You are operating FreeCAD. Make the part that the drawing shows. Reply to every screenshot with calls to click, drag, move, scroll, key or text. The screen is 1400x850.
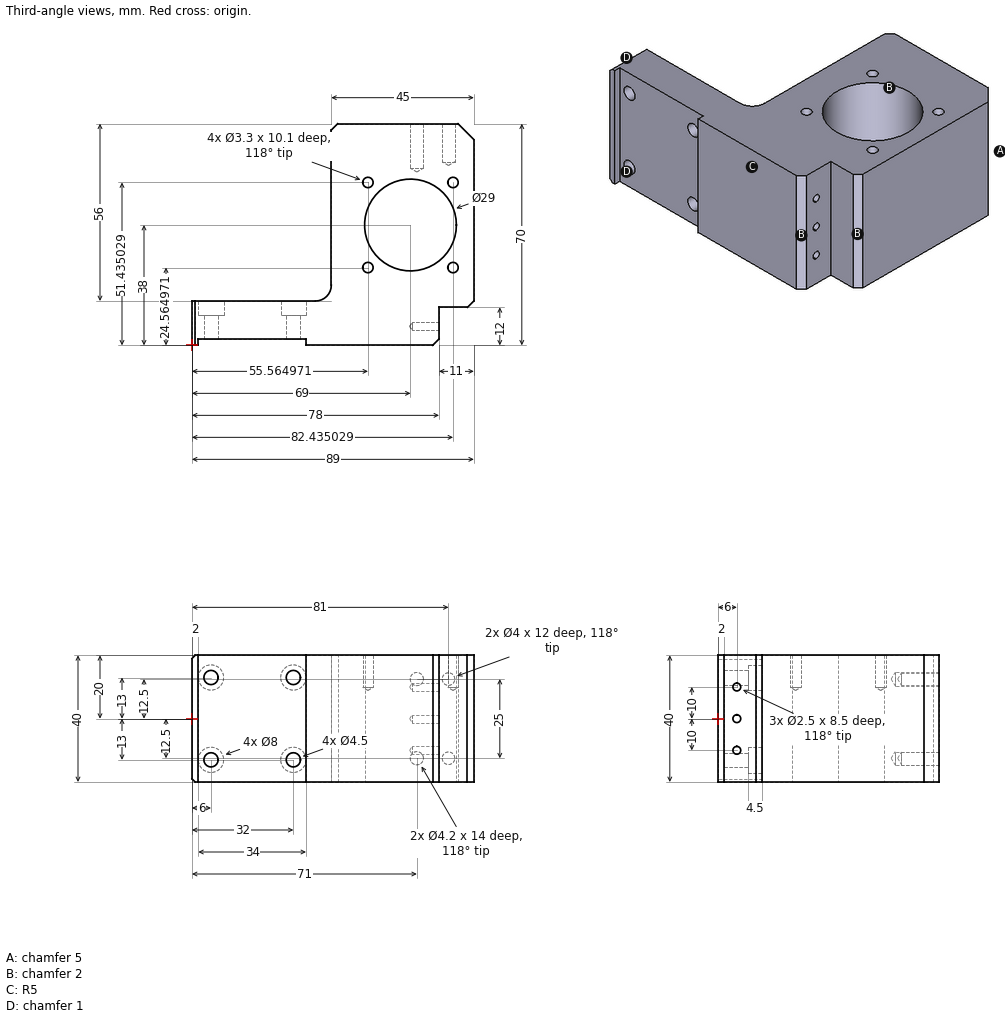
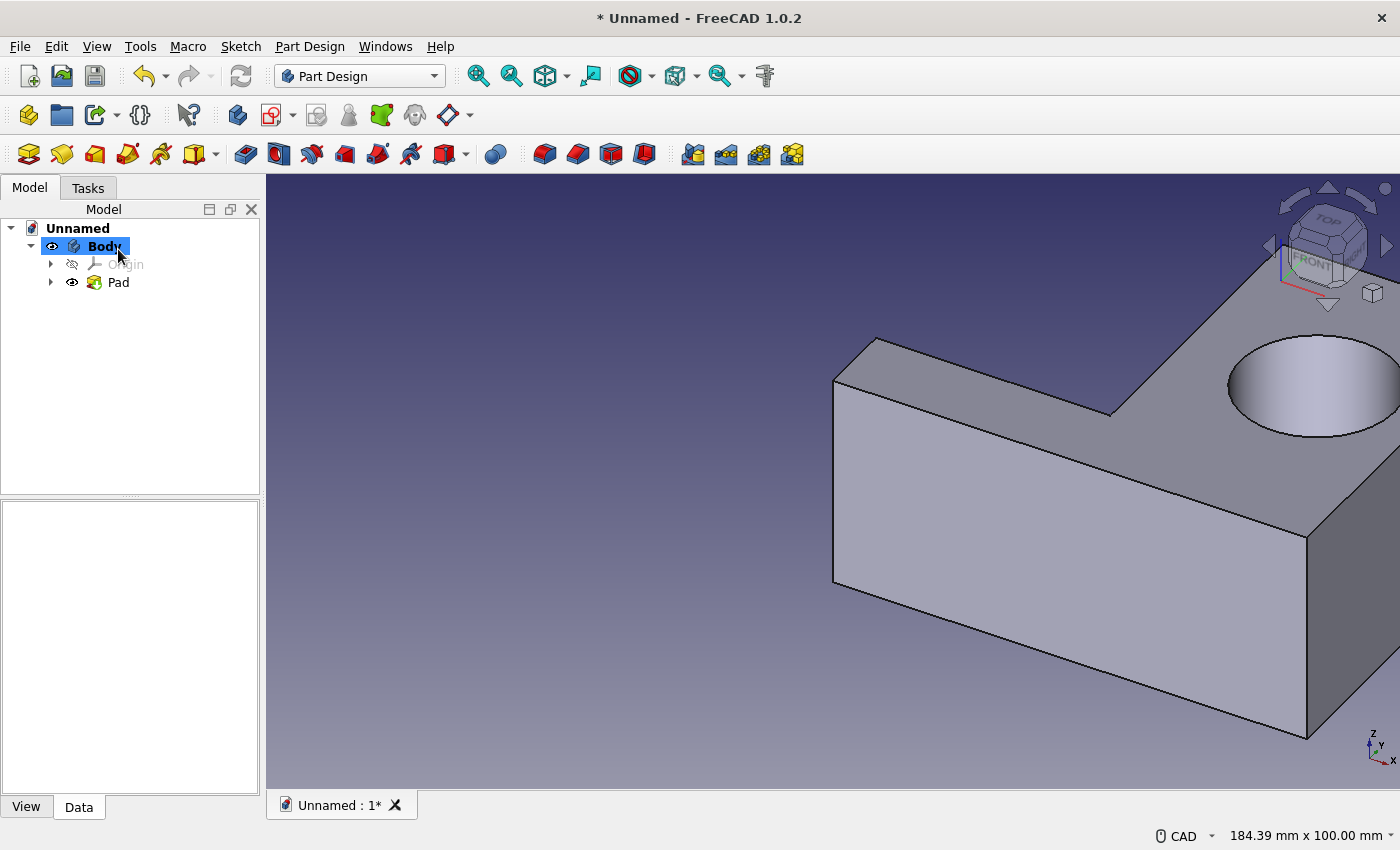
click(479, 76)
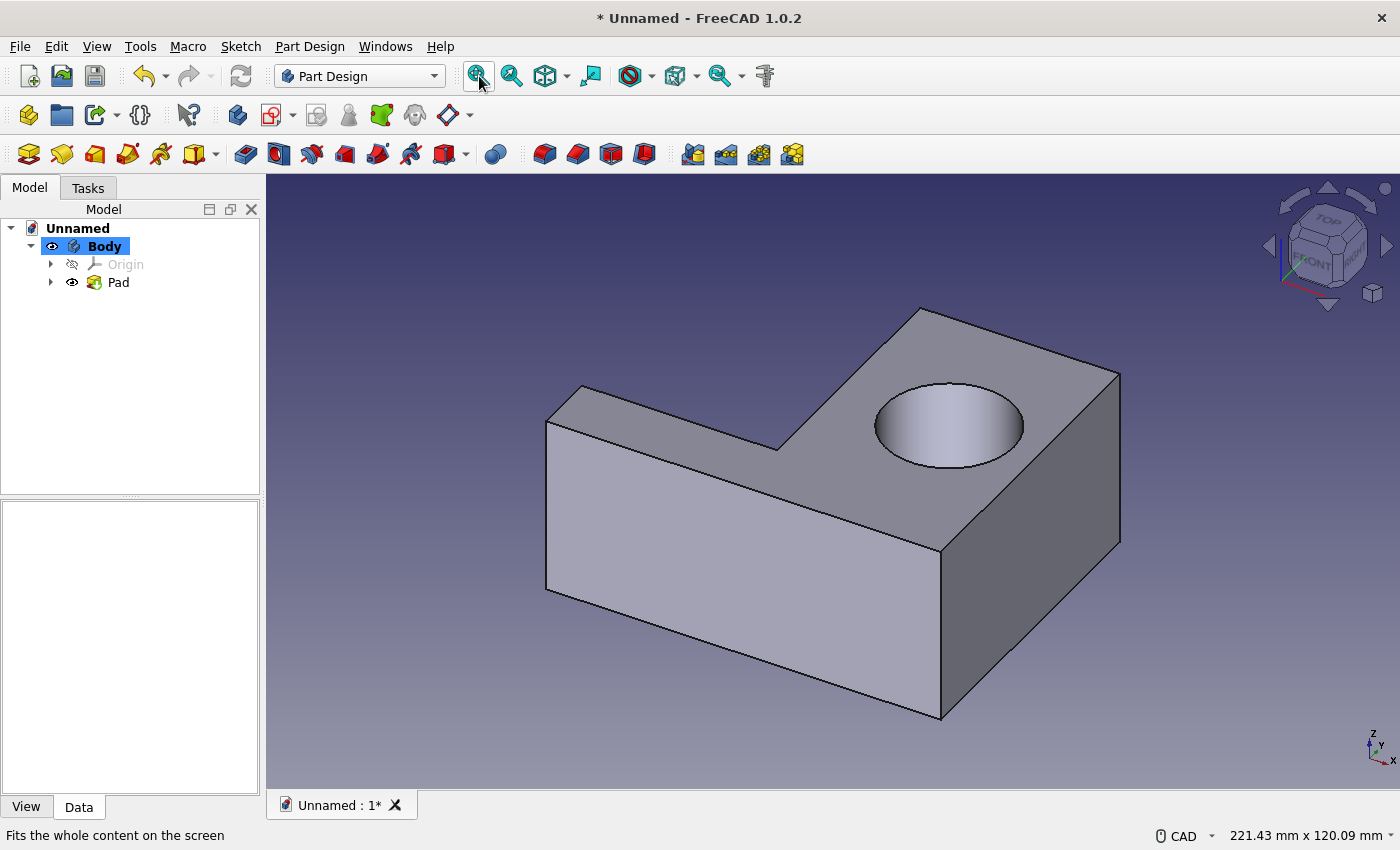
click(800, 588)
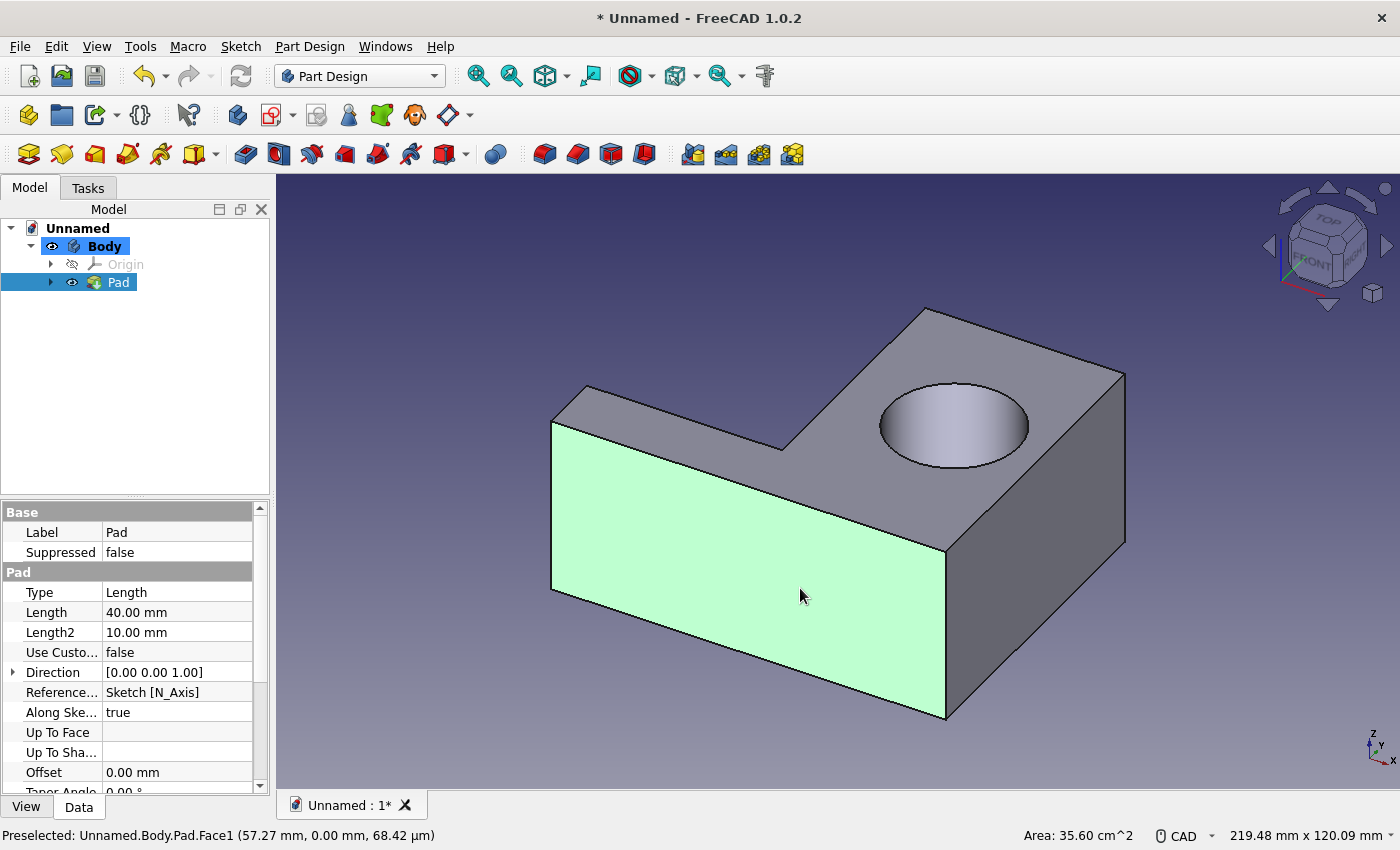
click(270, 116)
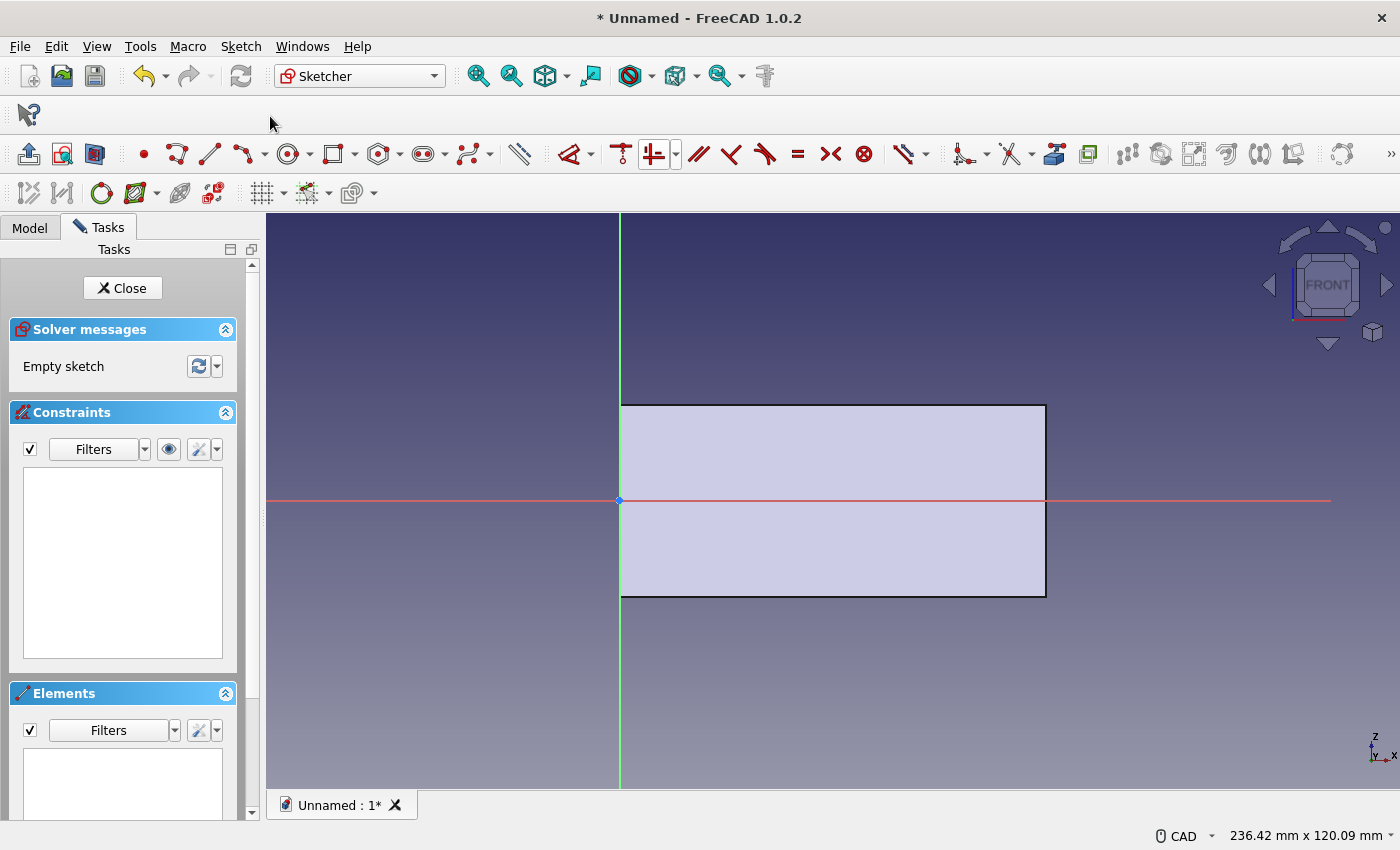
scroll(665, 501, up, 5)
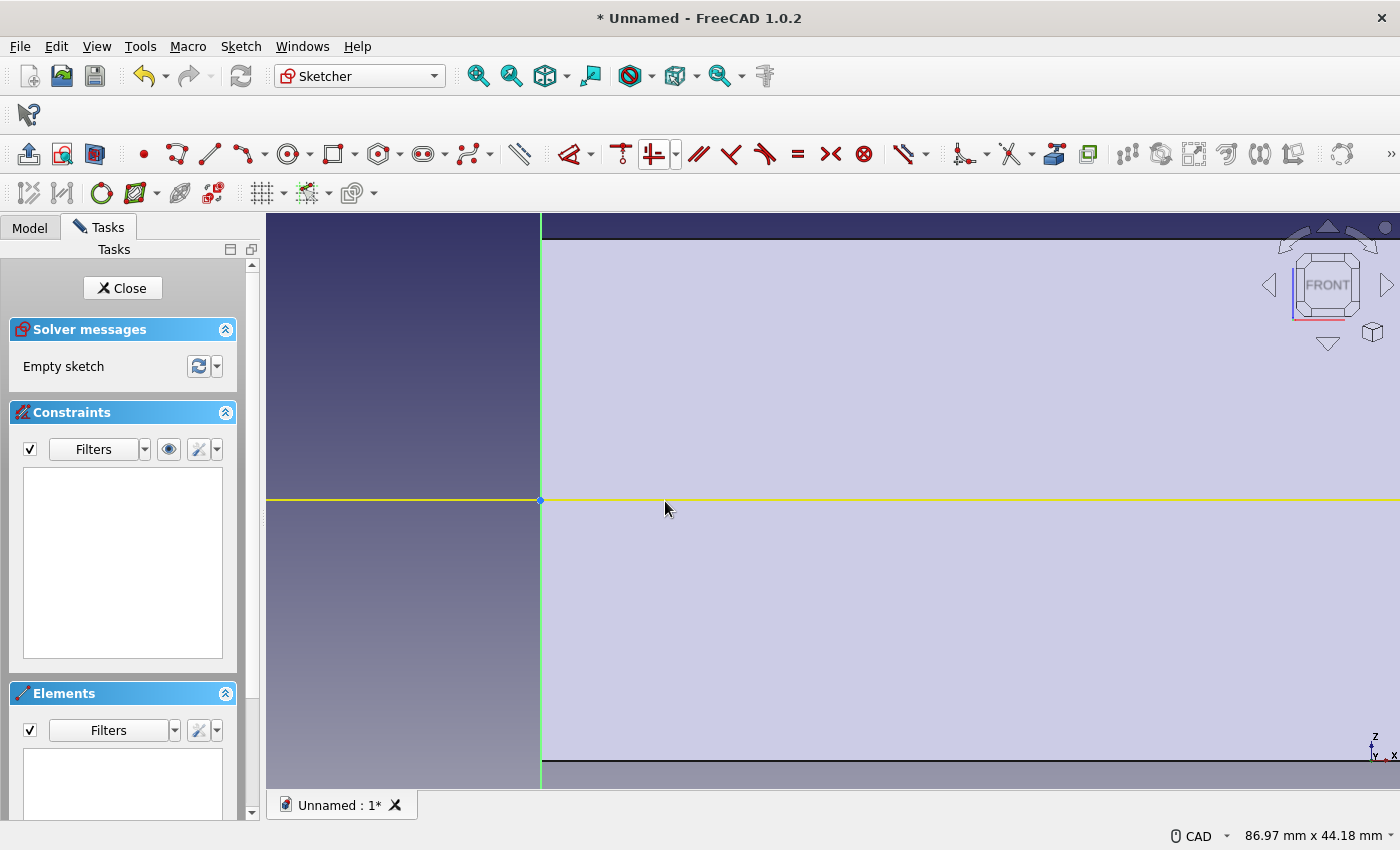
click(288, 154)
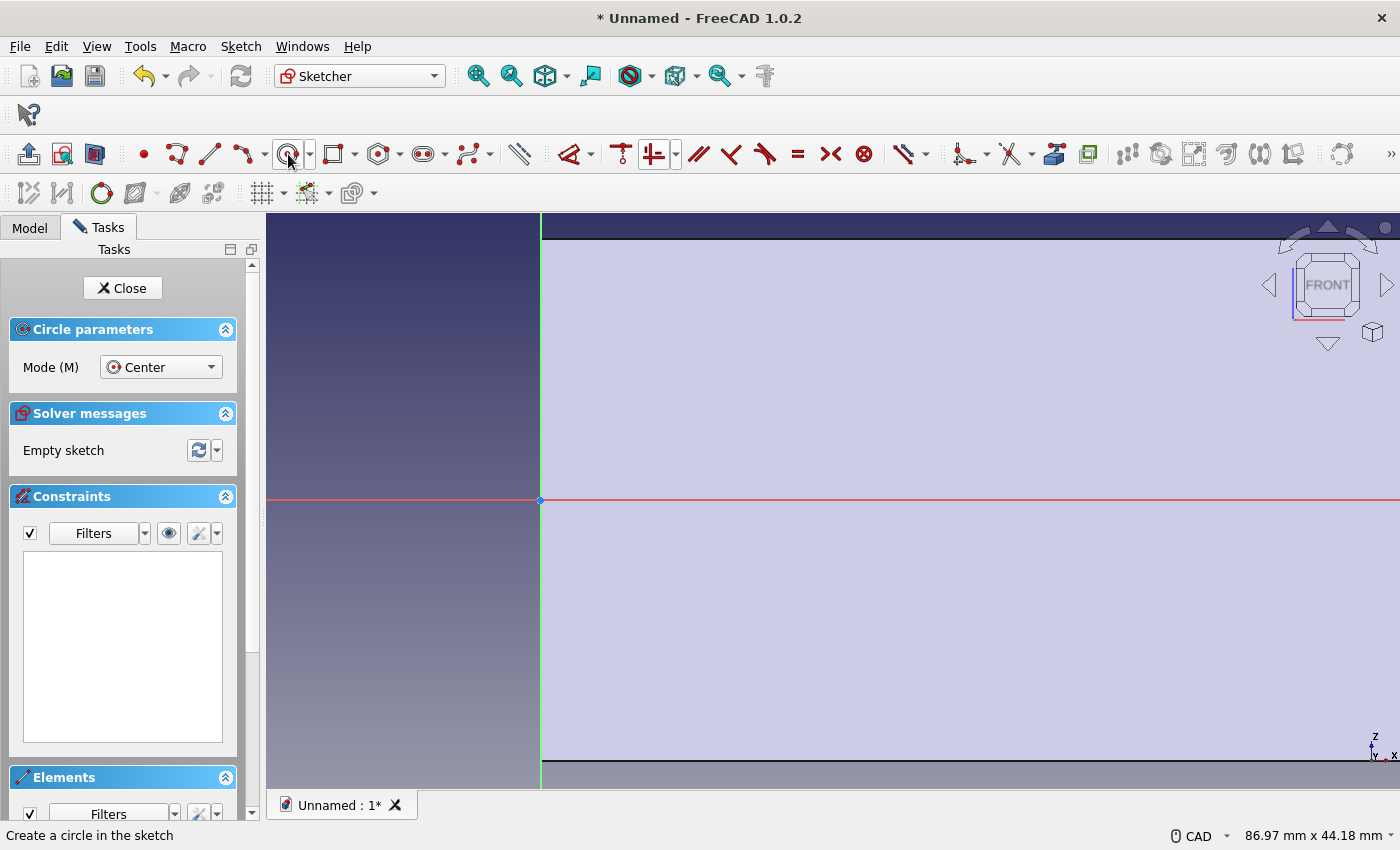
click(958, 670)
move(979, 649)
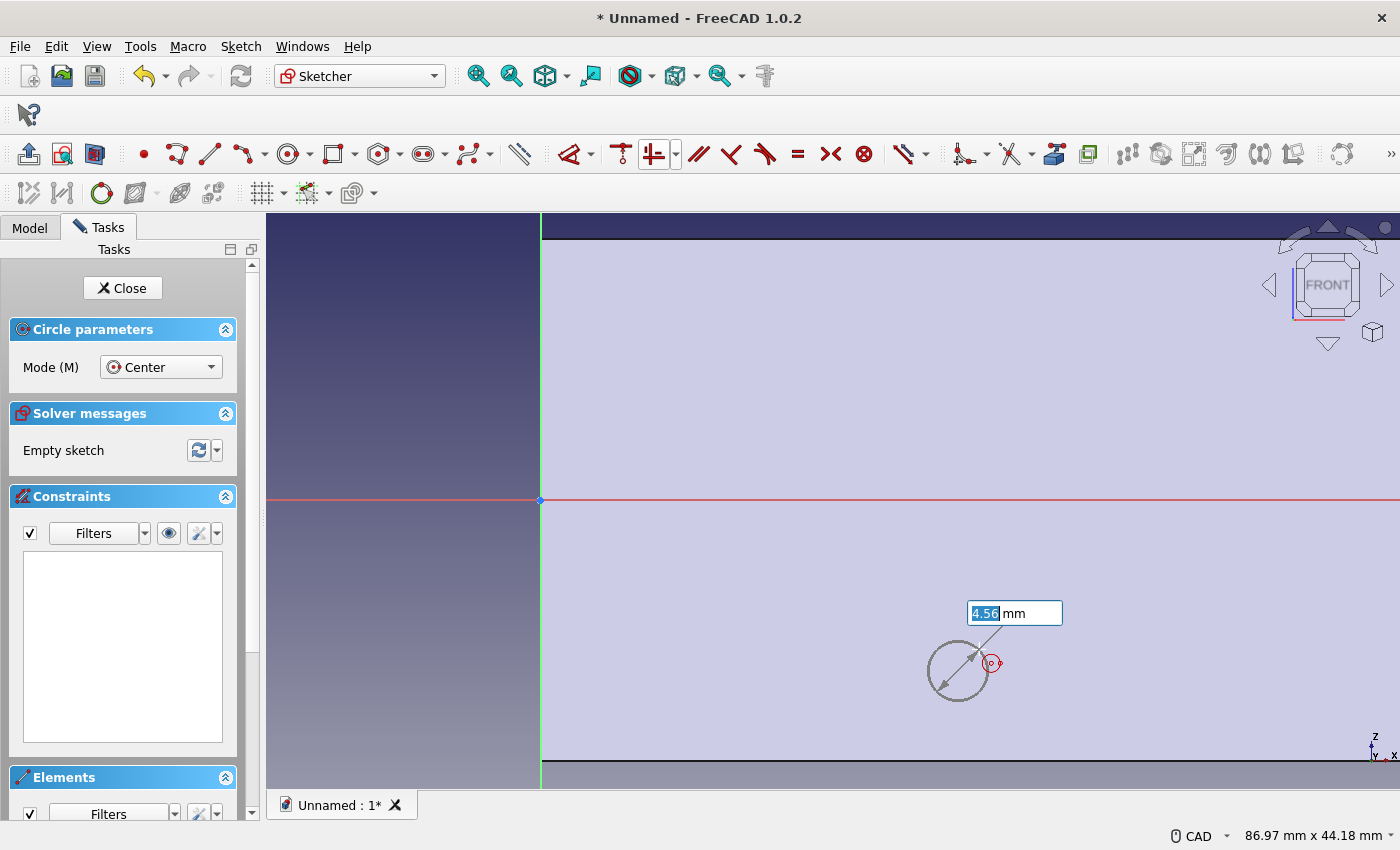
text(4.5)
key(Return)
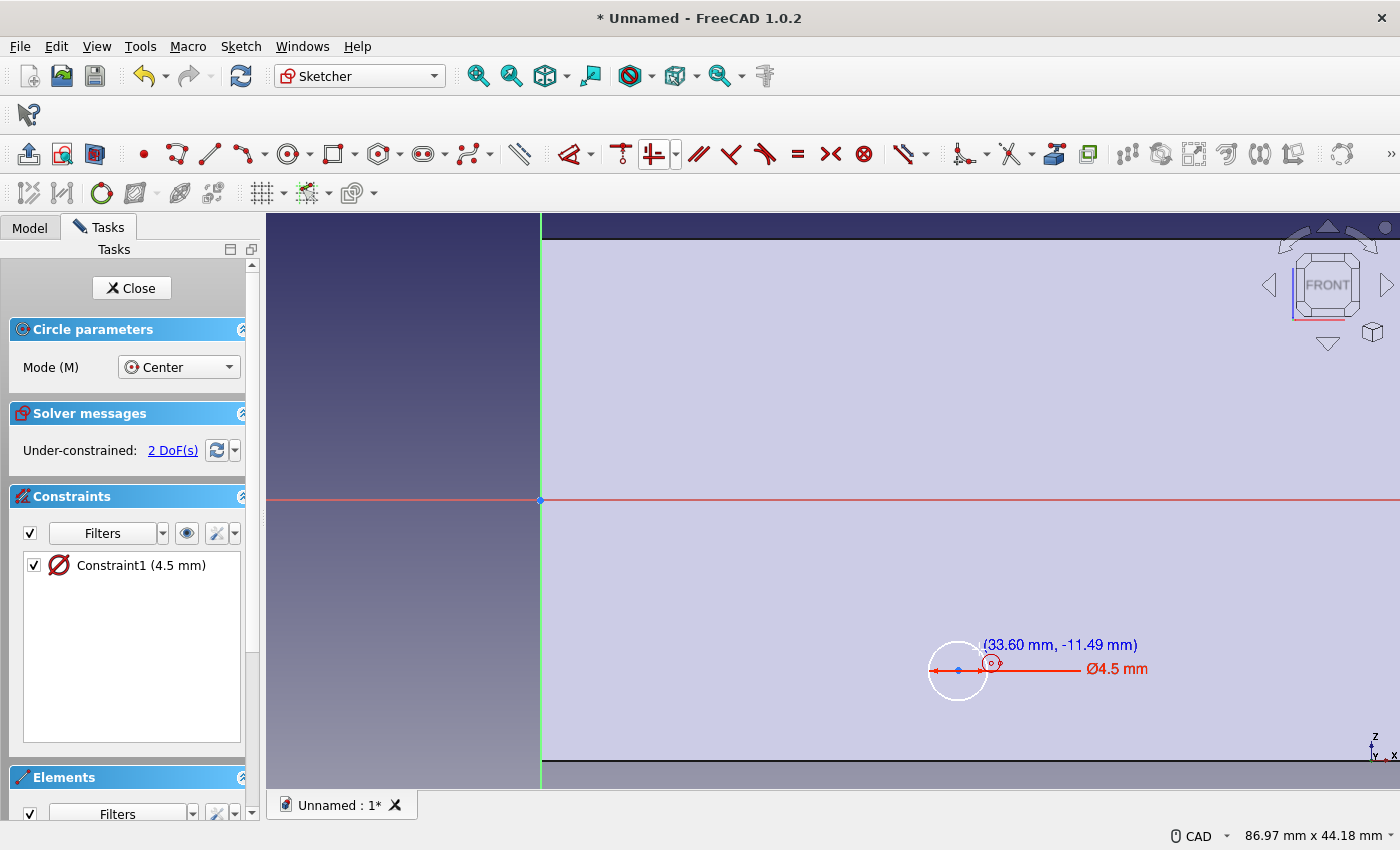
click(619, 670)
move(640, 649)